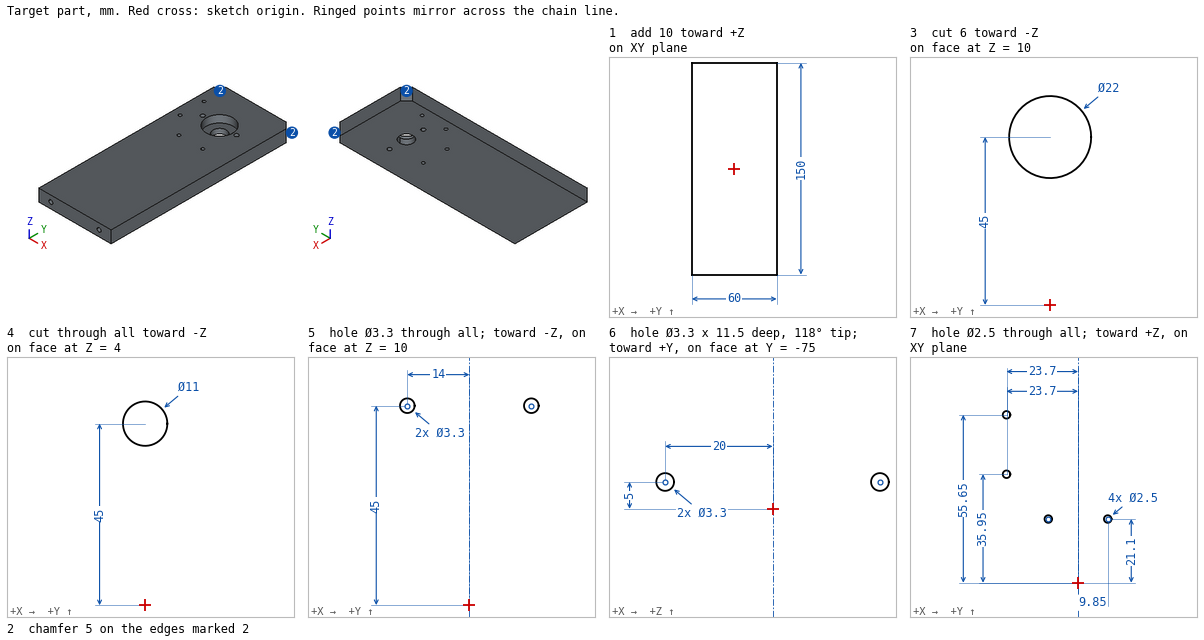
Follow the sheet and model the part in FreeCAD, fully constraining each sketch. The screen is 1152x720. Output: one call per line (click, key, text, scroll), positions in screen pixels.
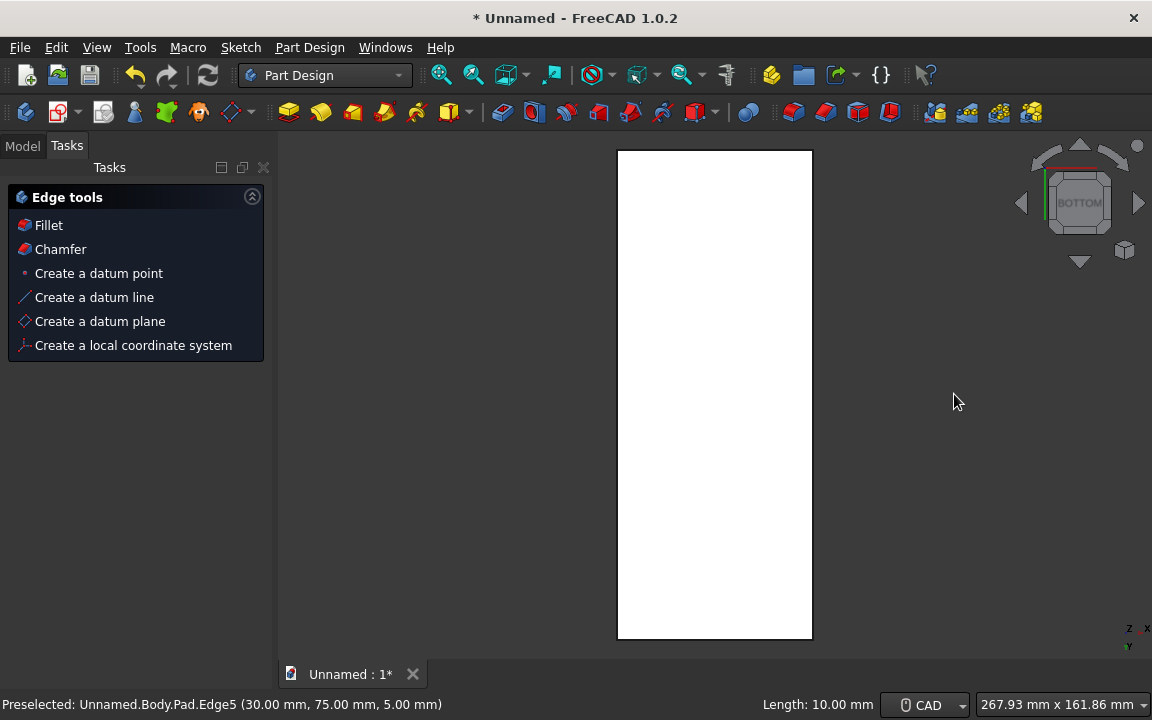
key(4)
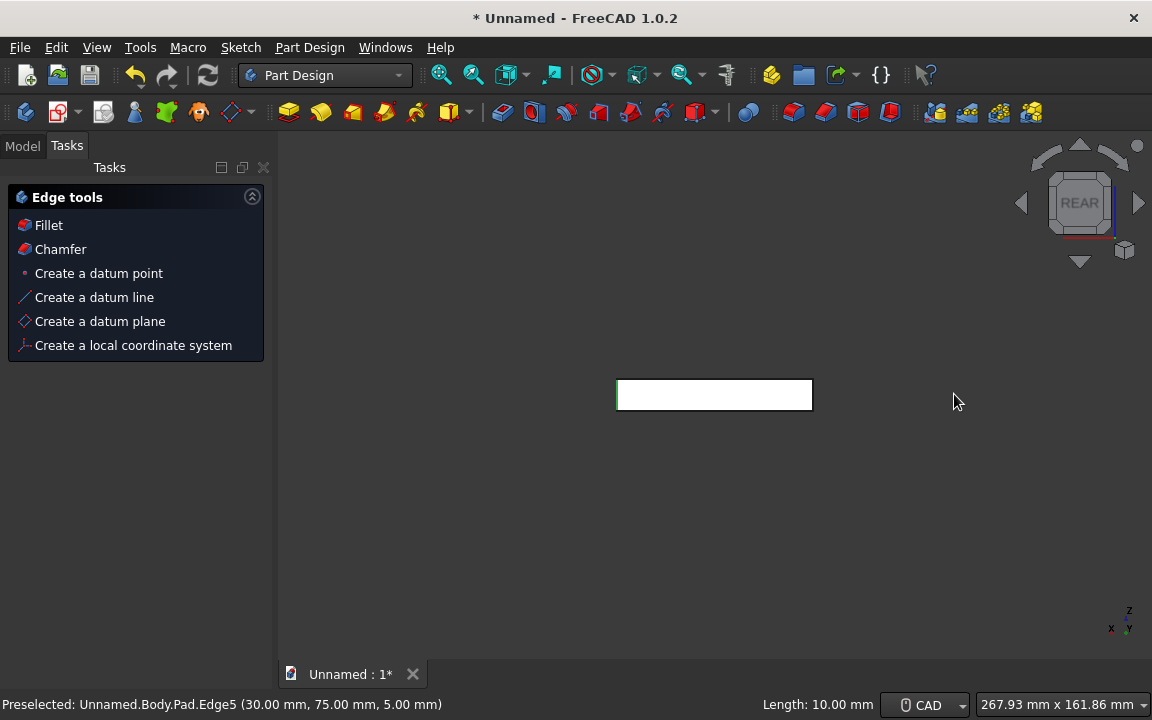
click(442, 76)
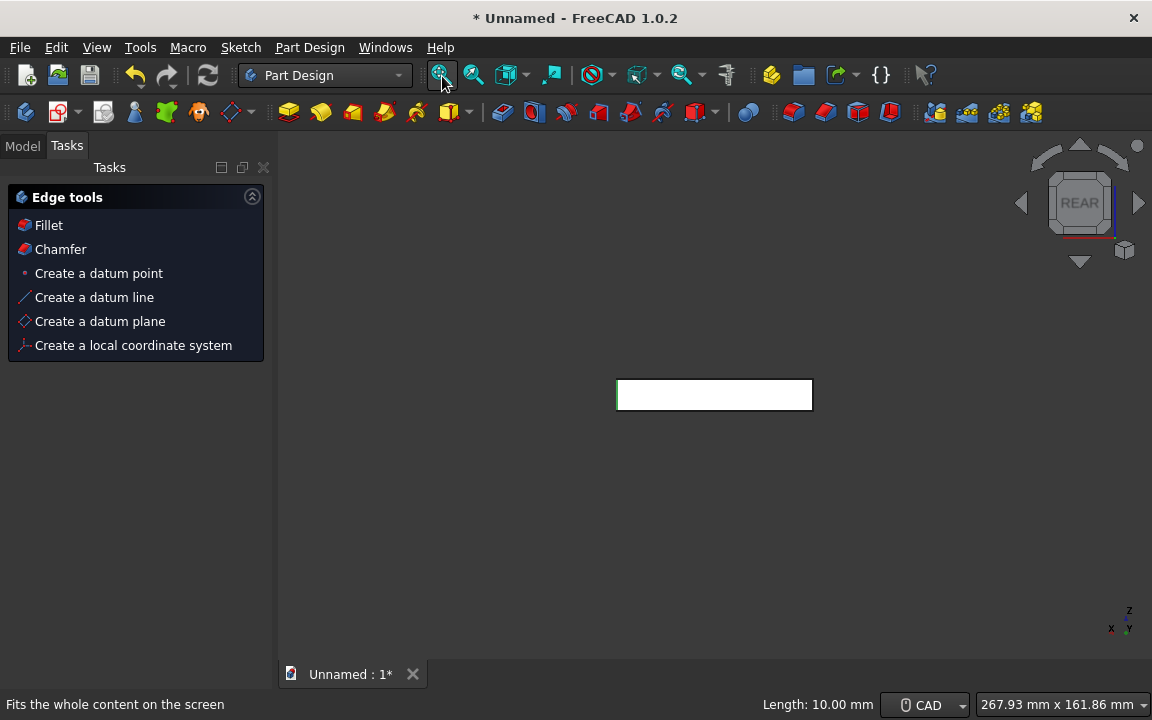
click(813, 394, ctrl)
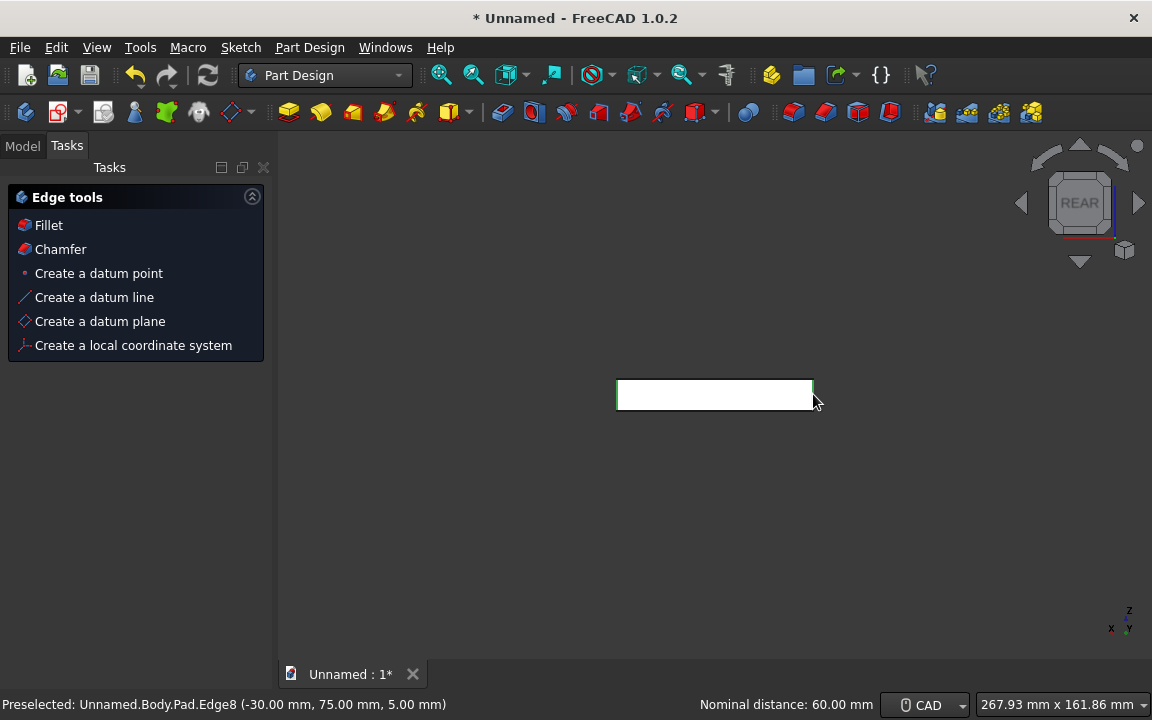
click(826, 112)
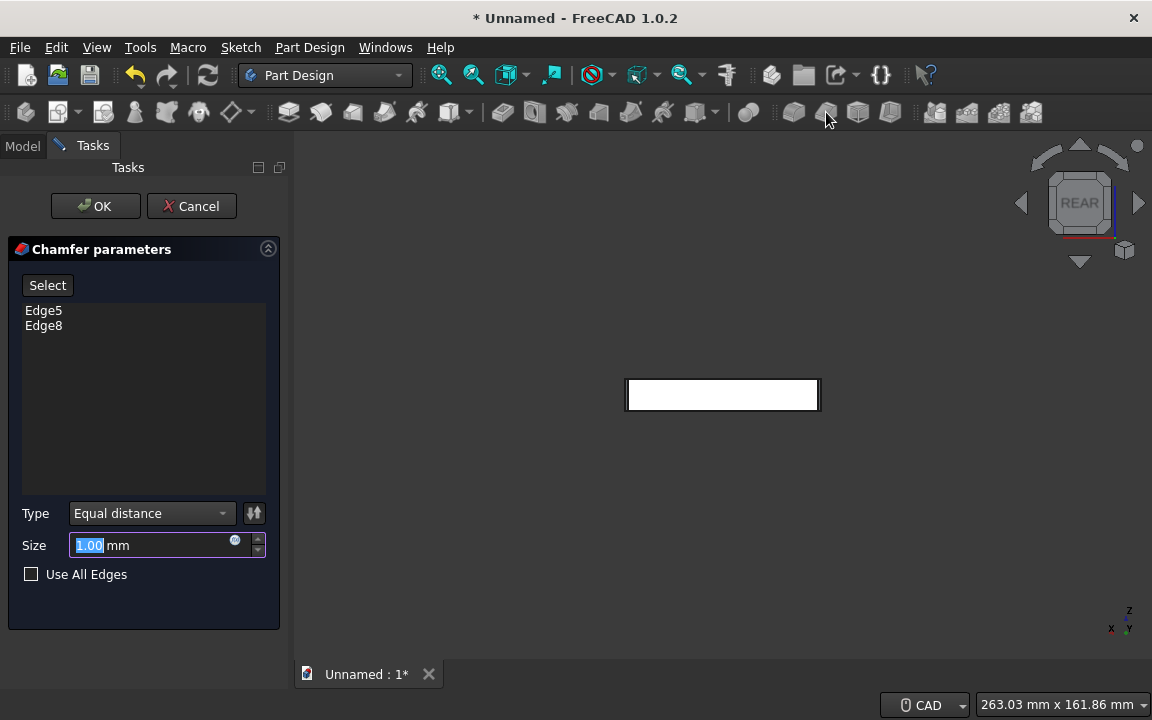
text(5)
key(Tab)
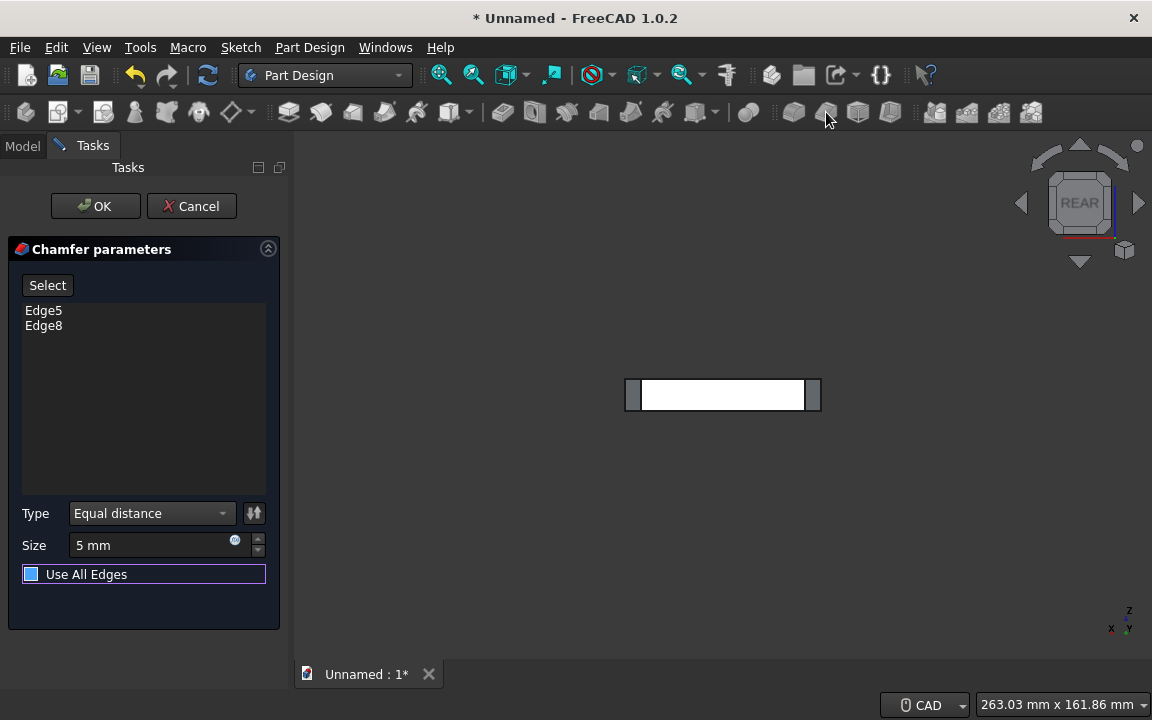
click(96, 206)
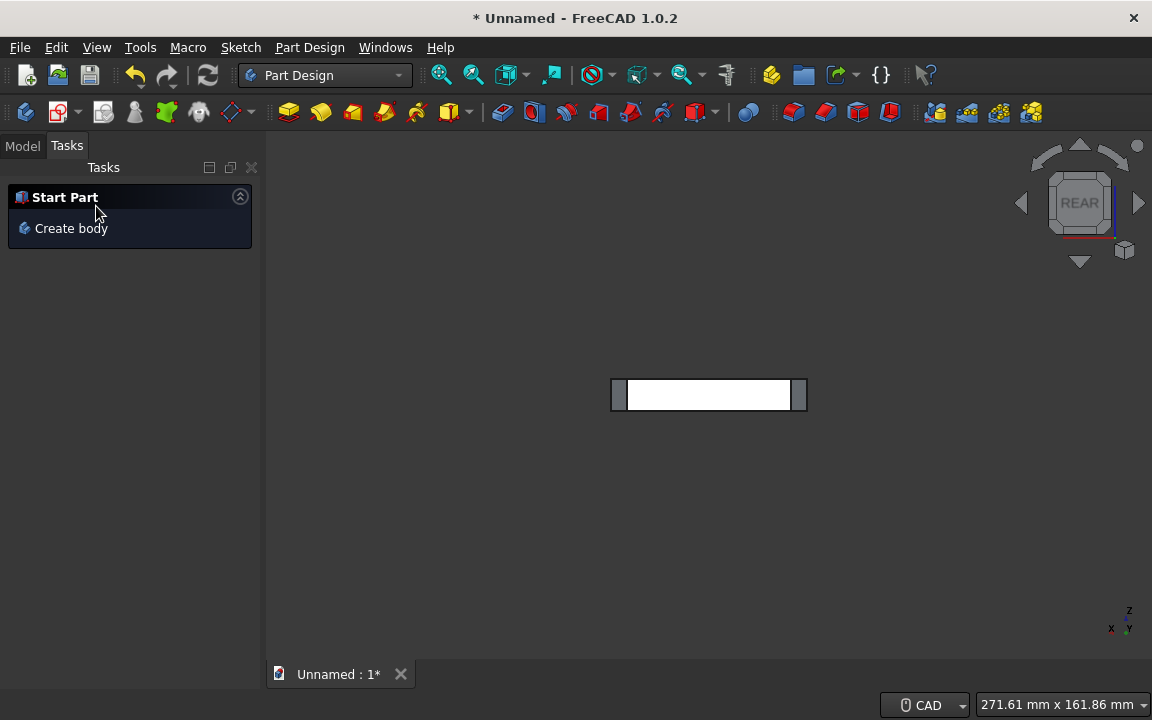
click(442, 76)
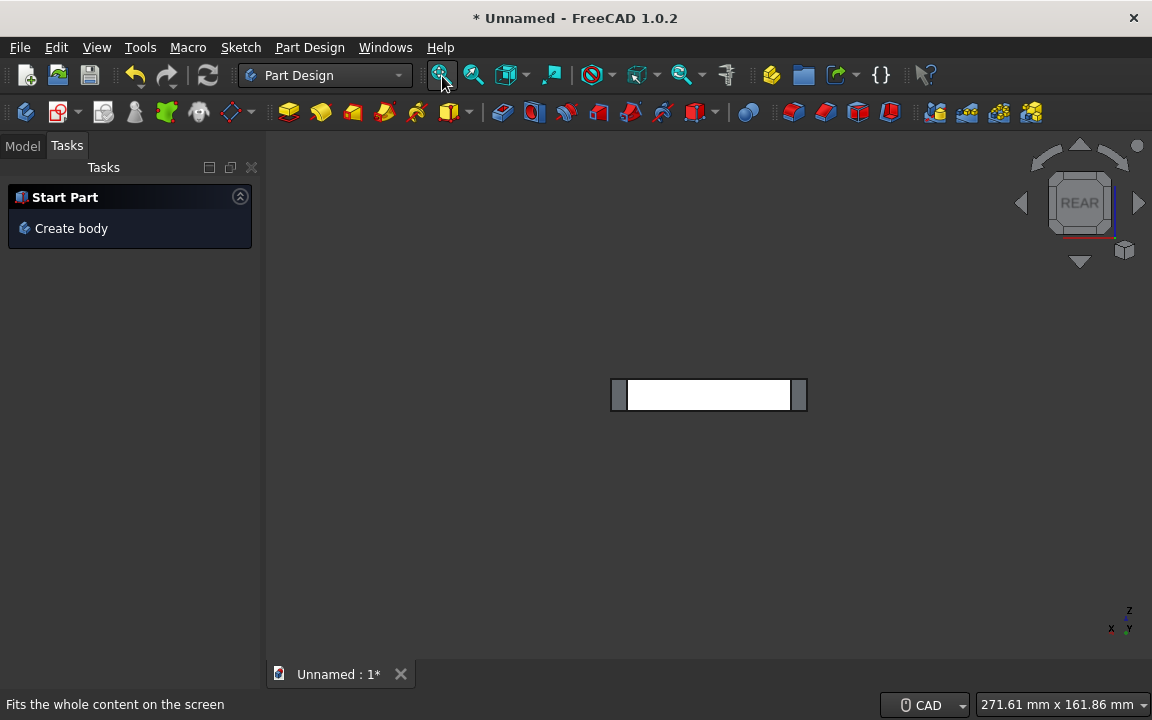
key(0)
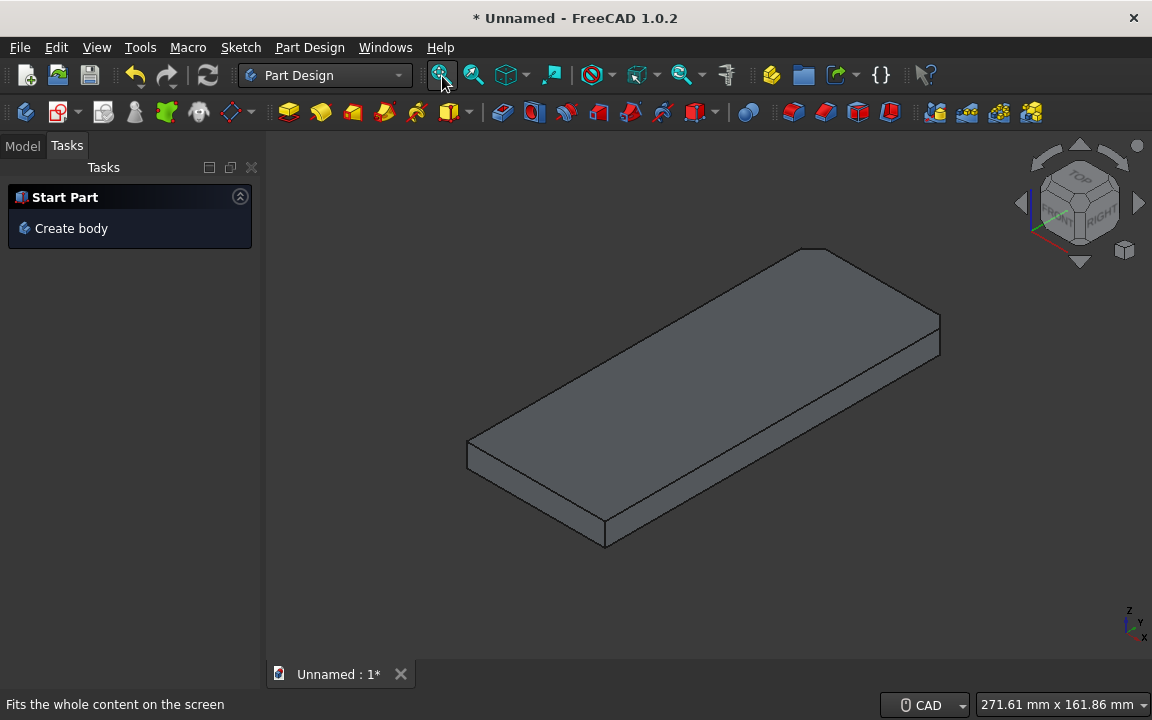
click(808, 324)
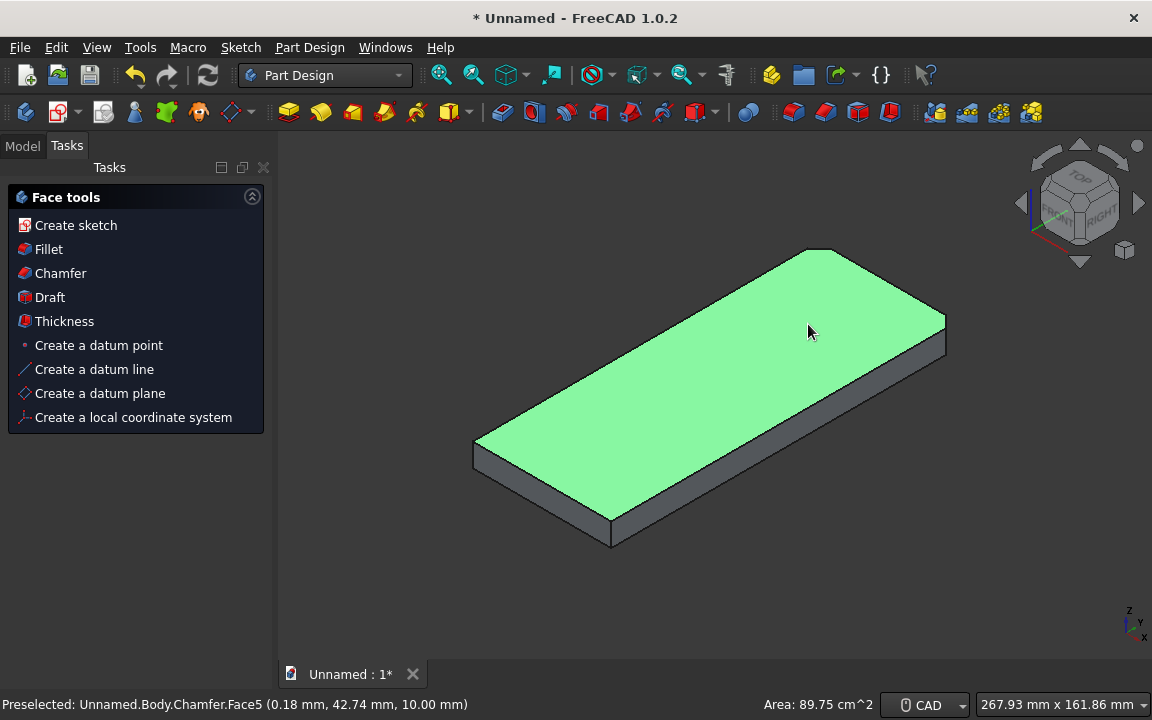
click(58, 112)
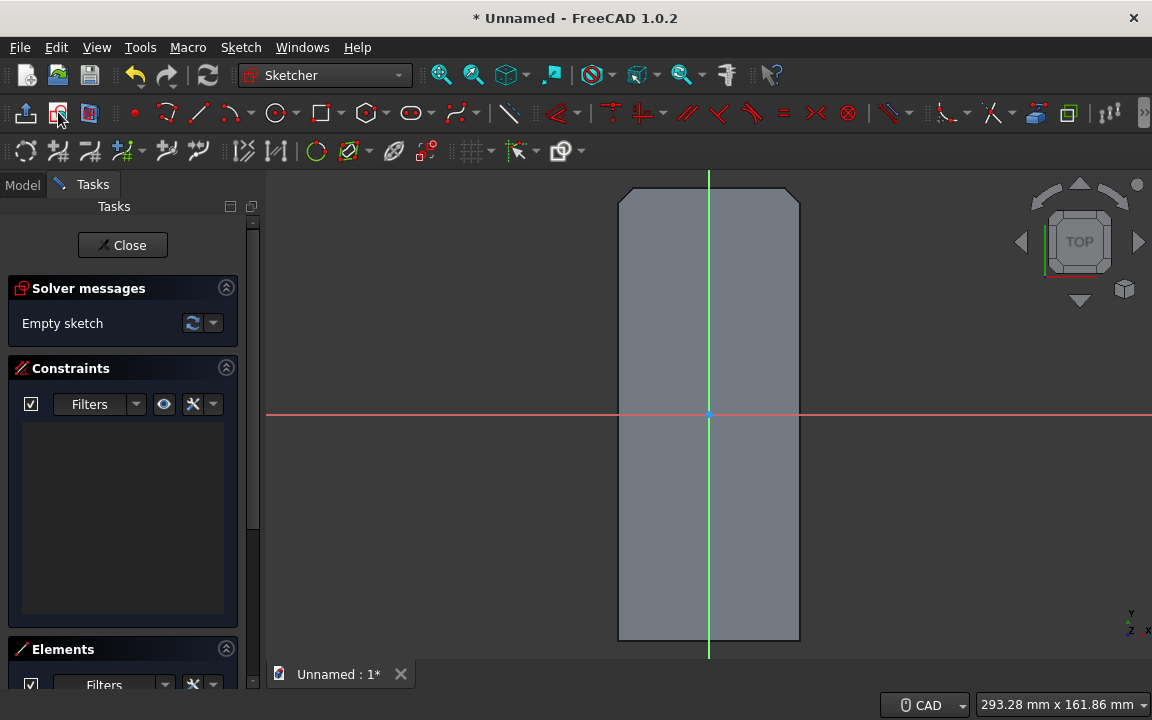
scroll(726, 244, up, 8)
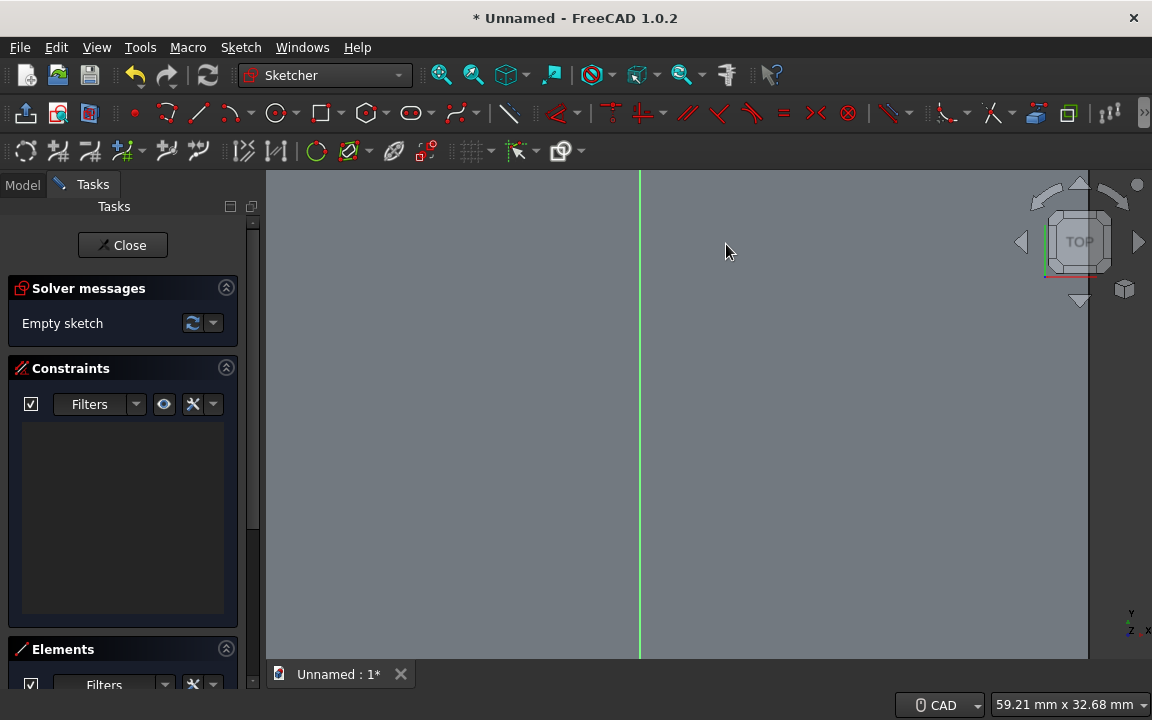
click(276, 114)